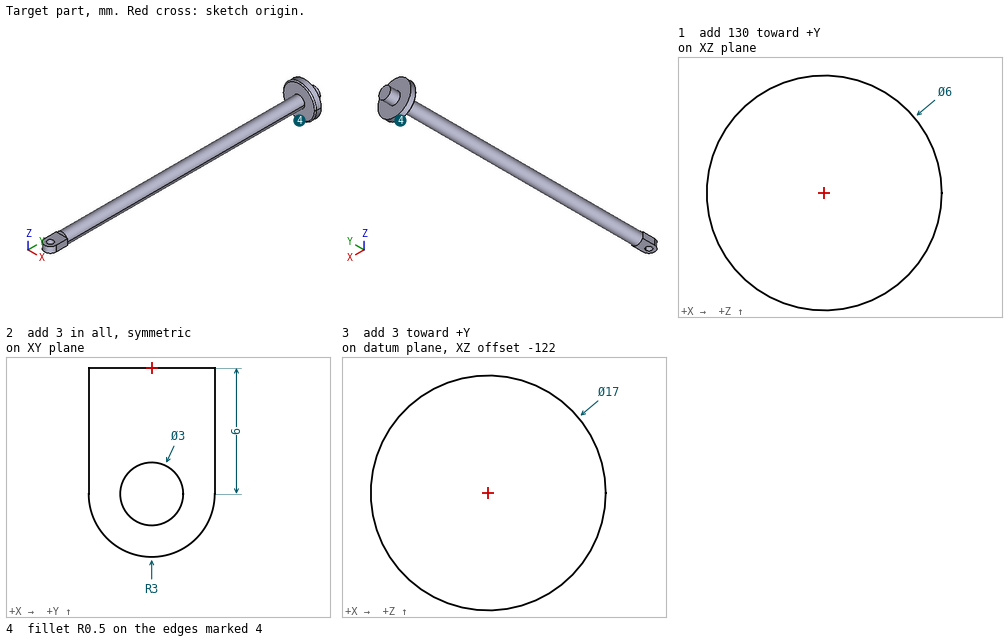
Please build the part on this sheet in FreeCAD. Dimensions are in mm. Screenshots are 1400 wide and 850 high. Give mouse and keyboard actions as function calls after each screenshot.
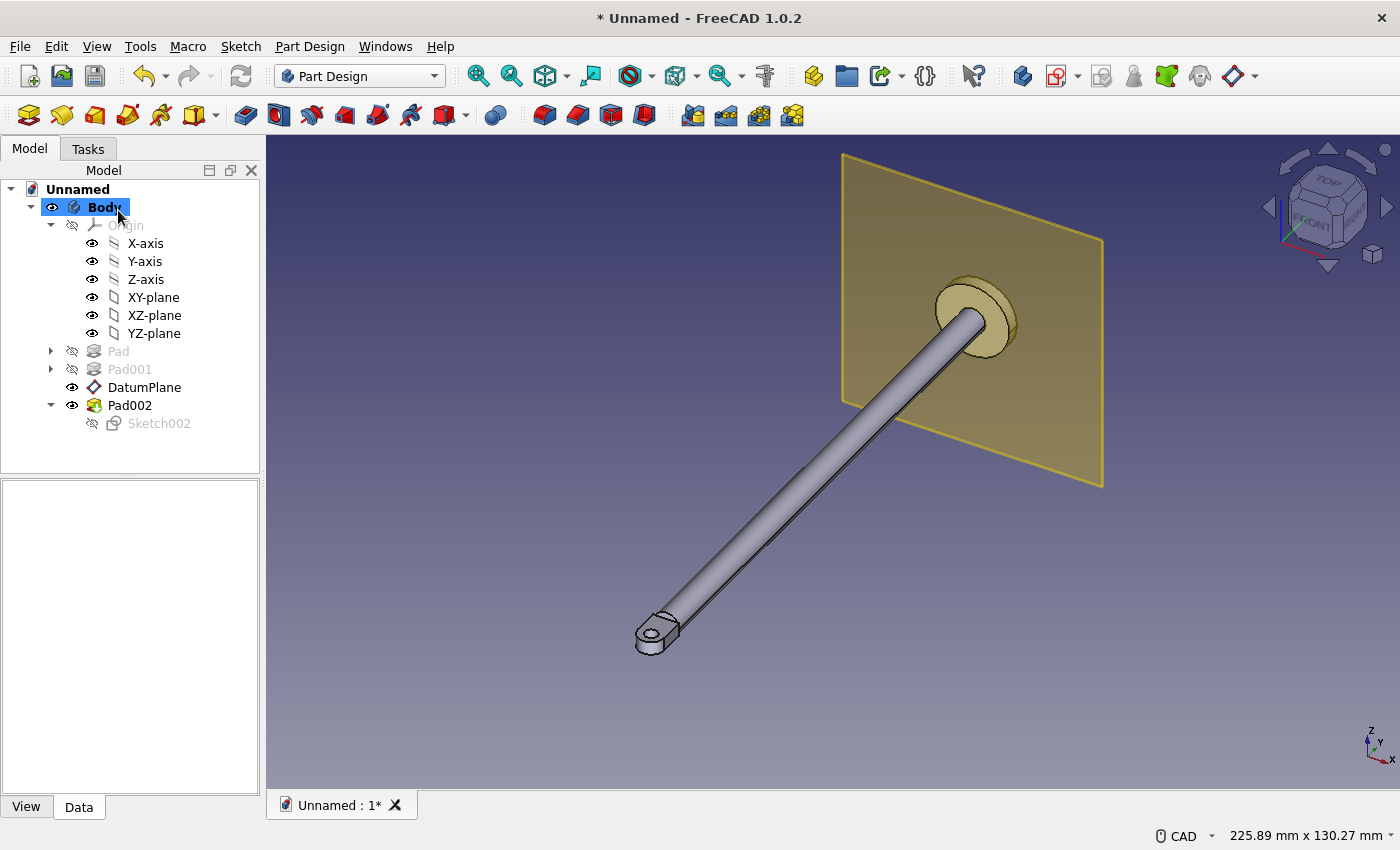
click(117, 387)
key(space)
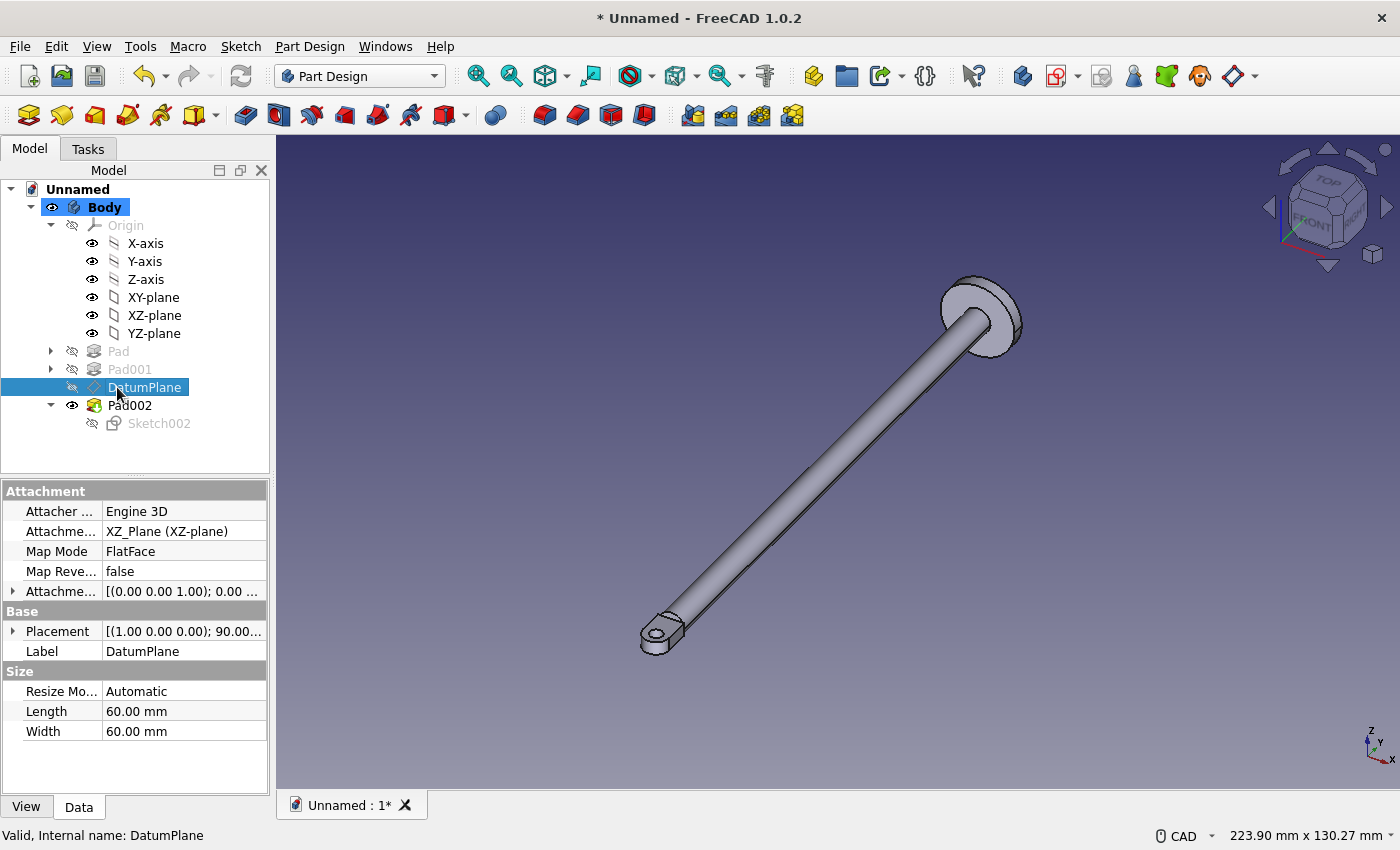
click(948, 289)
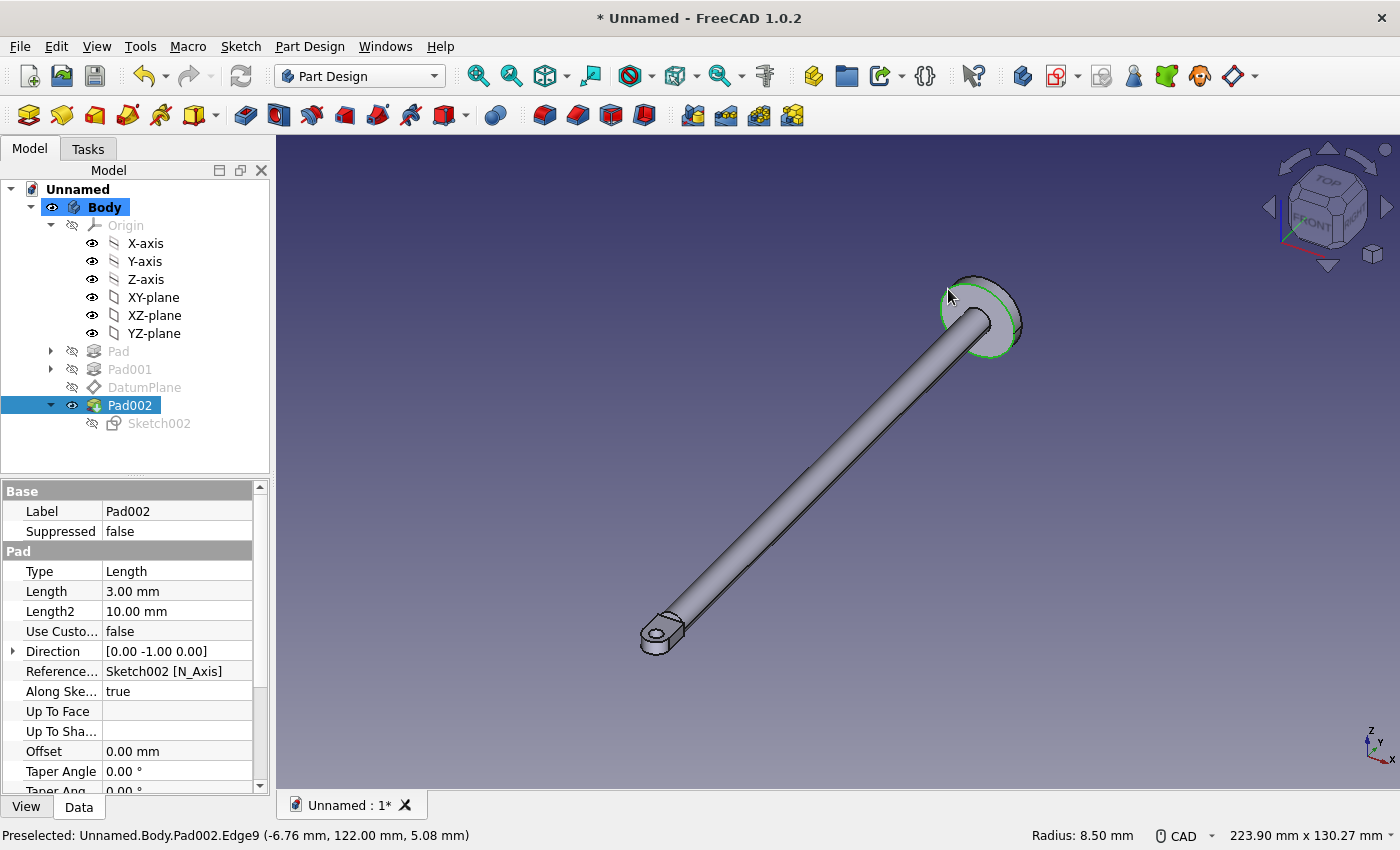
click(545, 116)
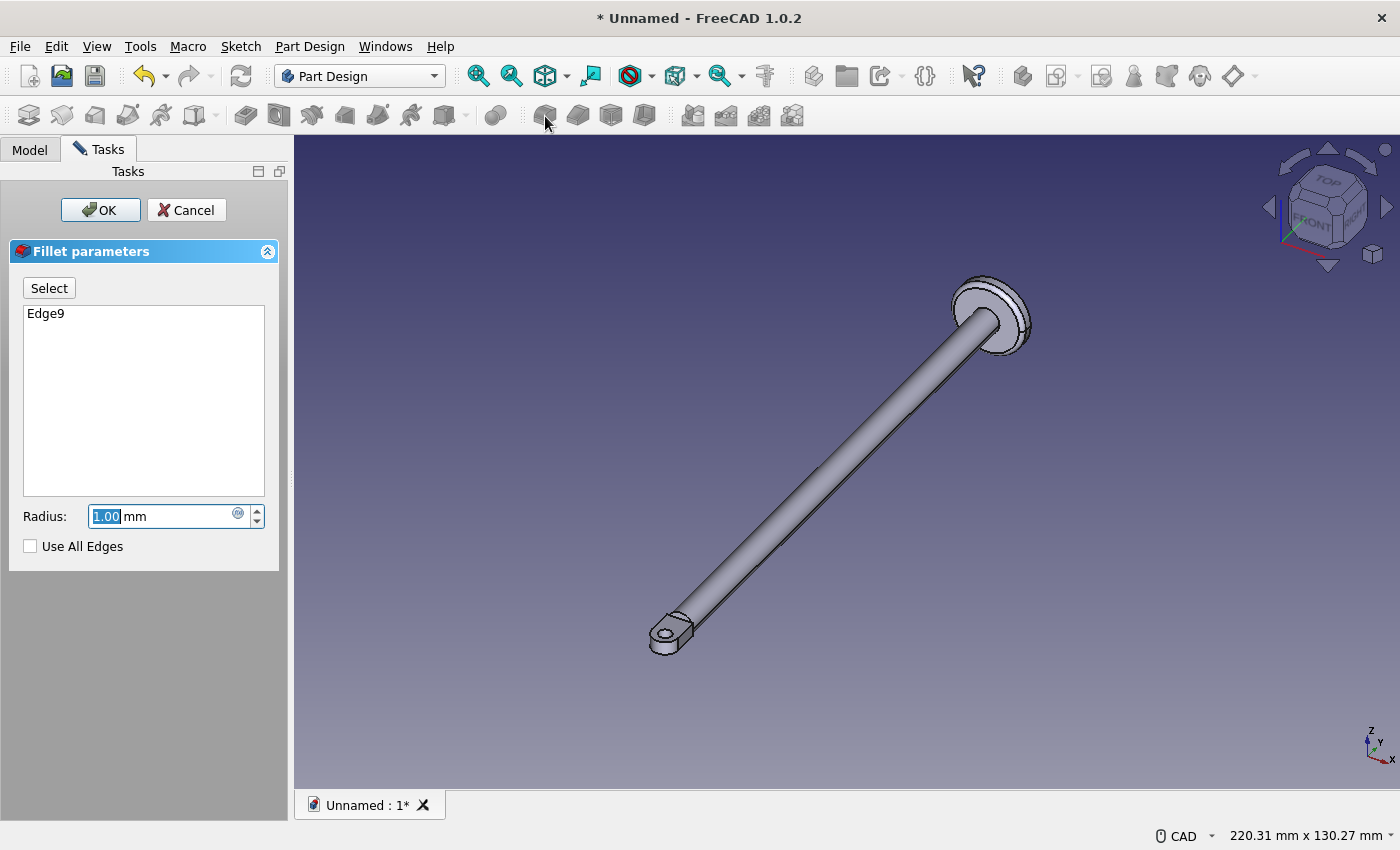
text(0.5)
key(Tab)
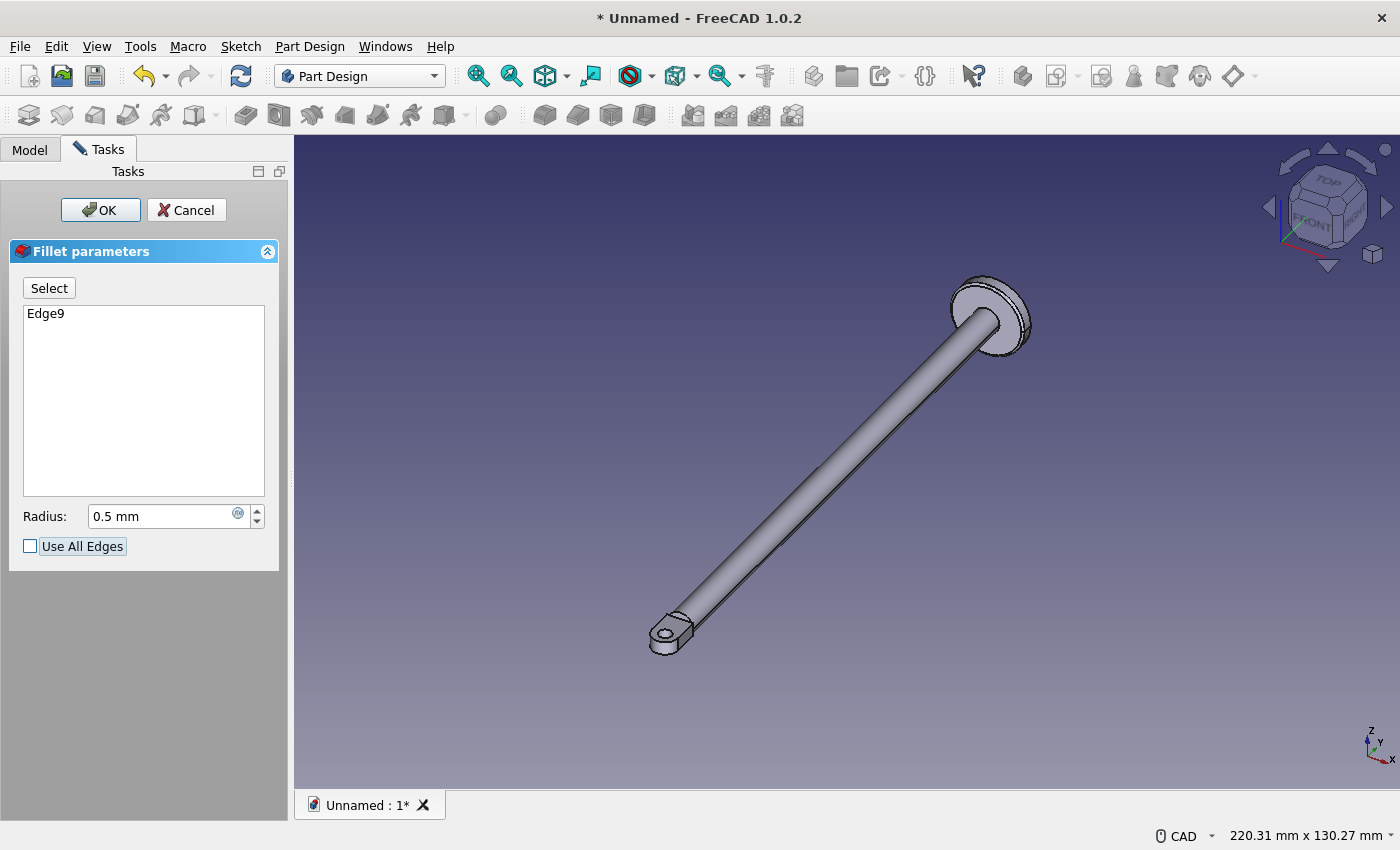
click(101, 210)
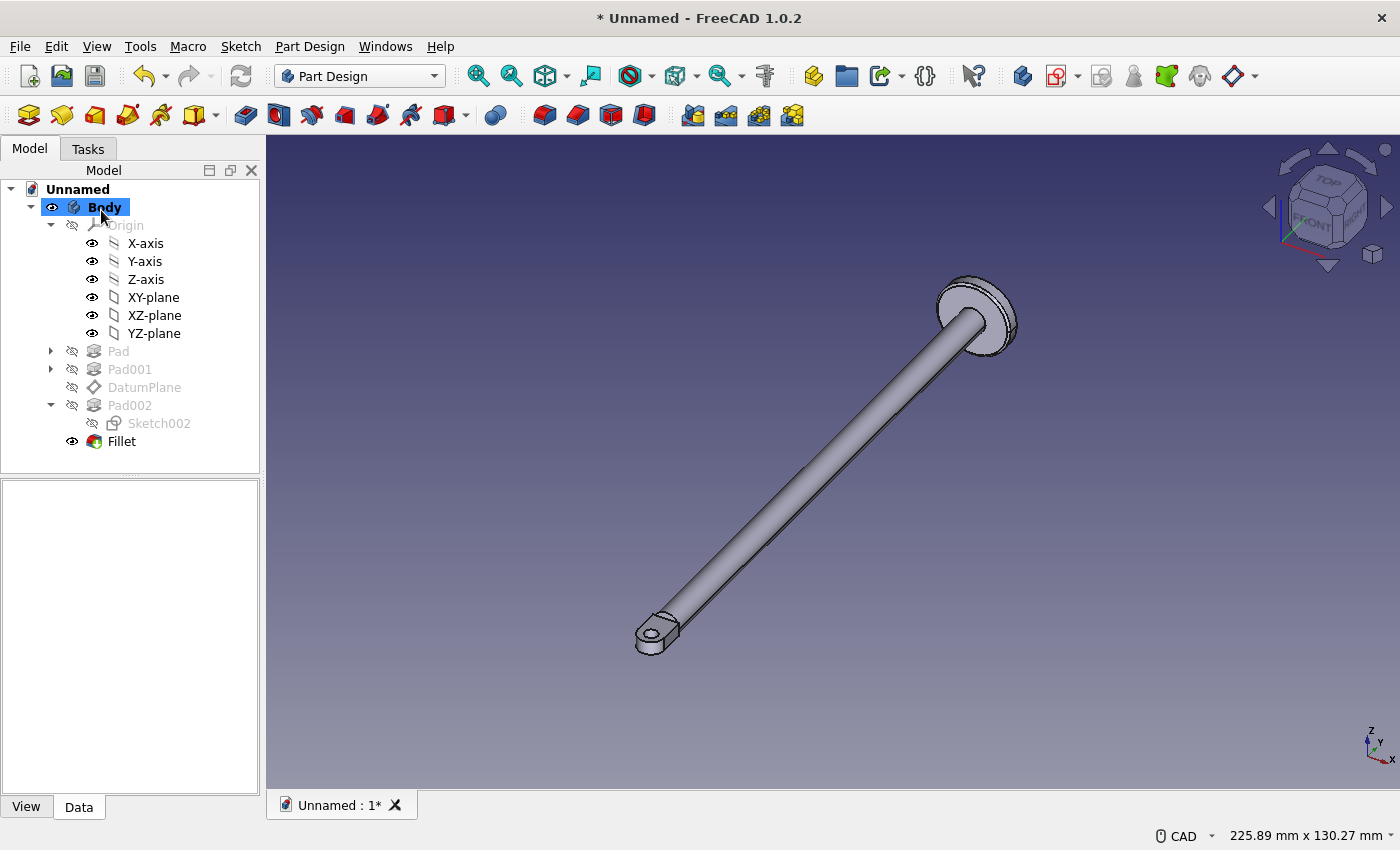
key(0)